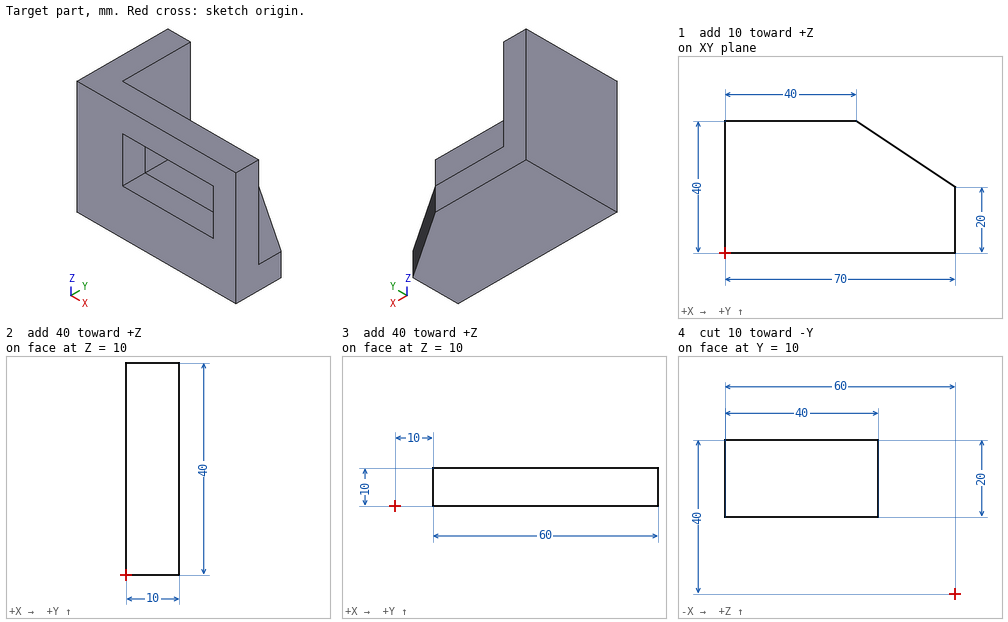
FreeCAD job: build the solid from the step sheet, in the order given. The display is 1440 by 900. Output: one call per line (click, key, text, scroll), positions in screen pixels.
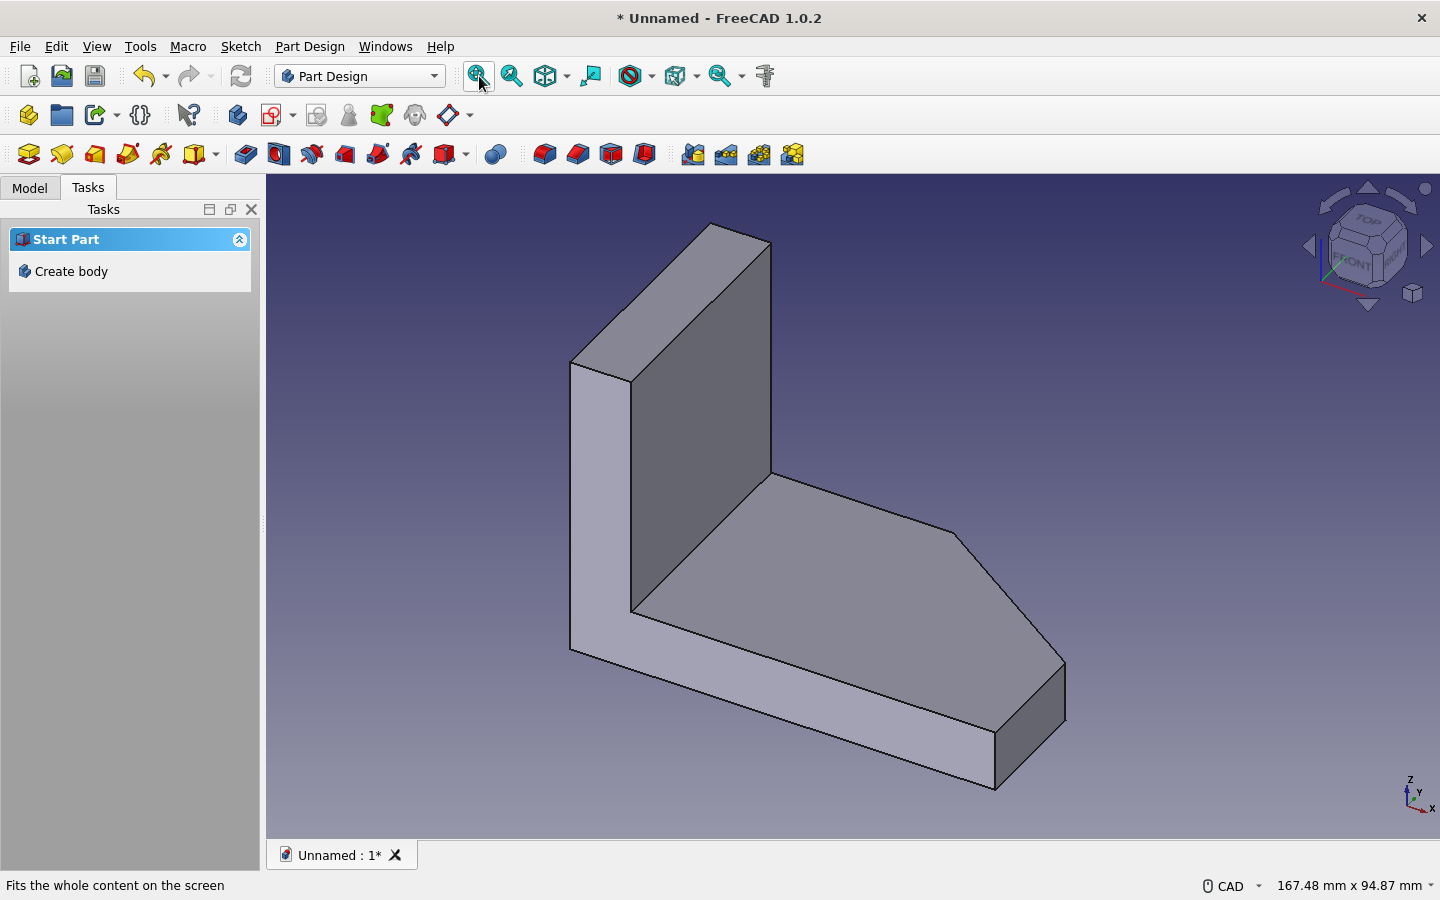
click(831, 584)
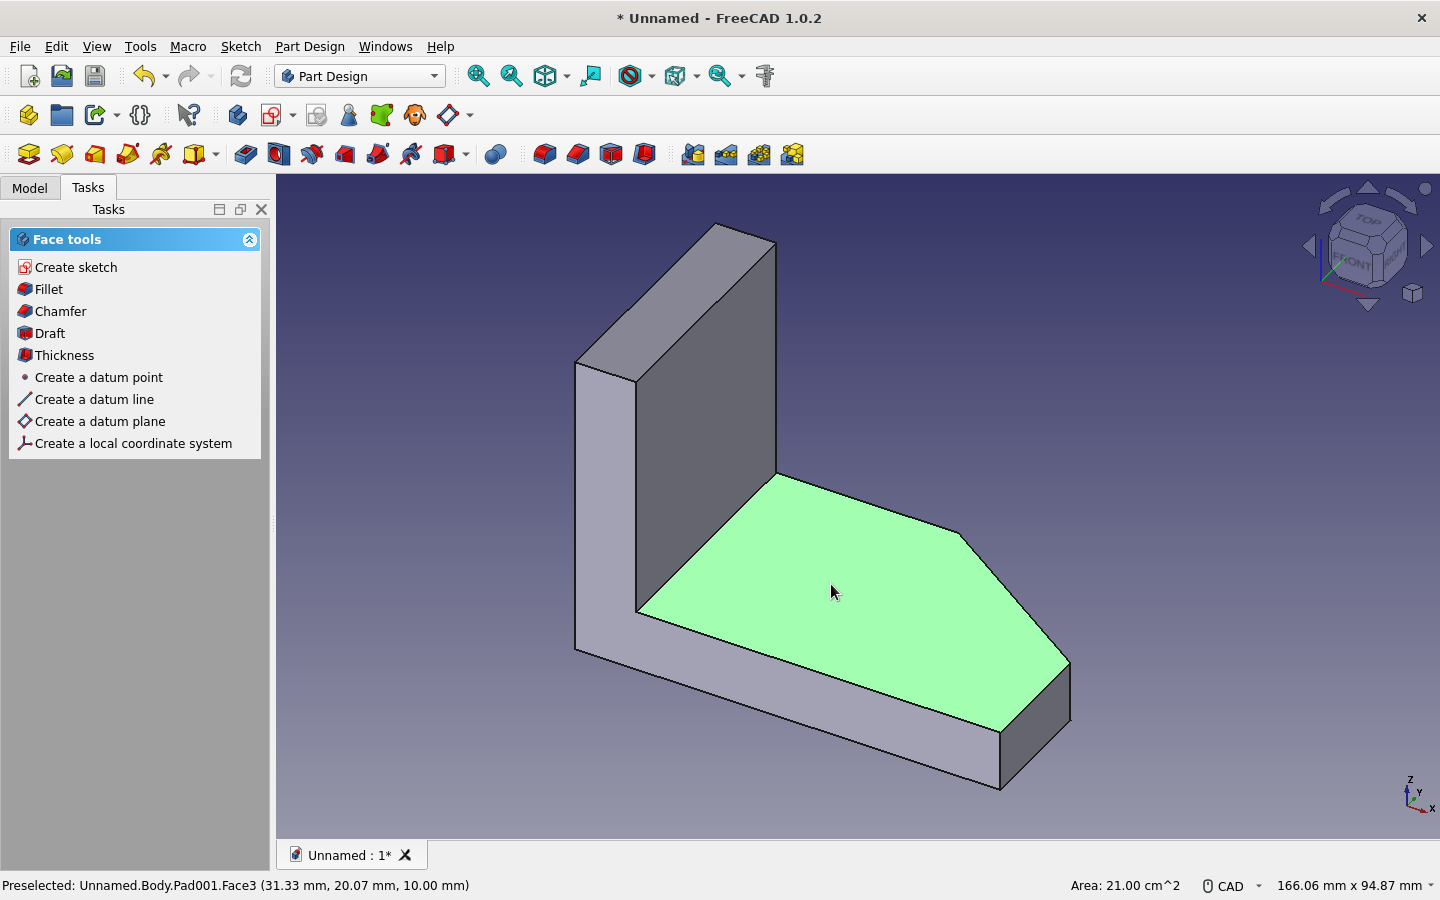
click(270, 116)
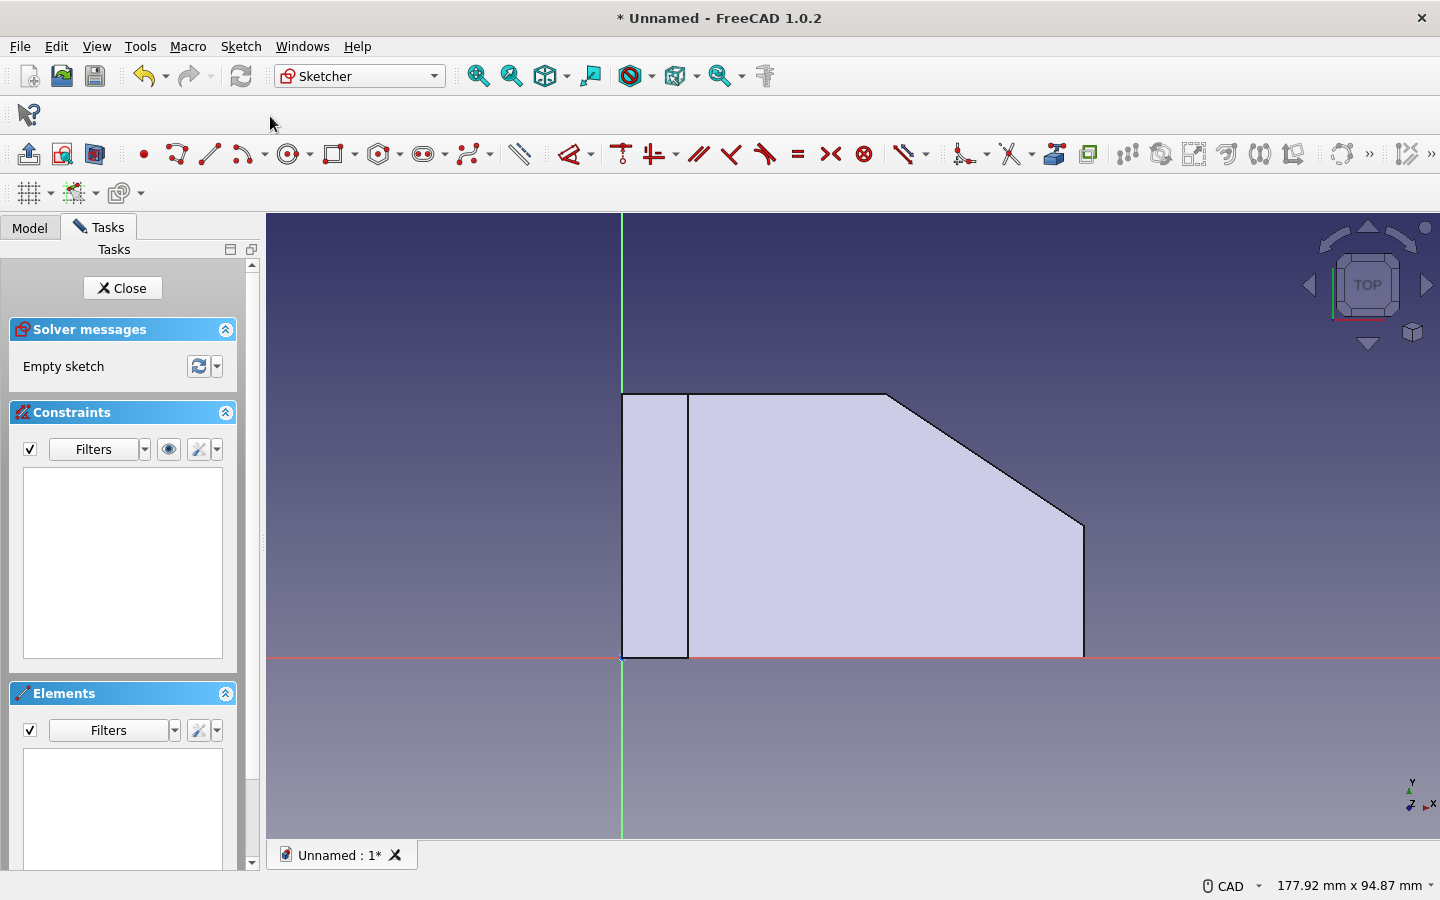
scroll(992, 811, up, 2)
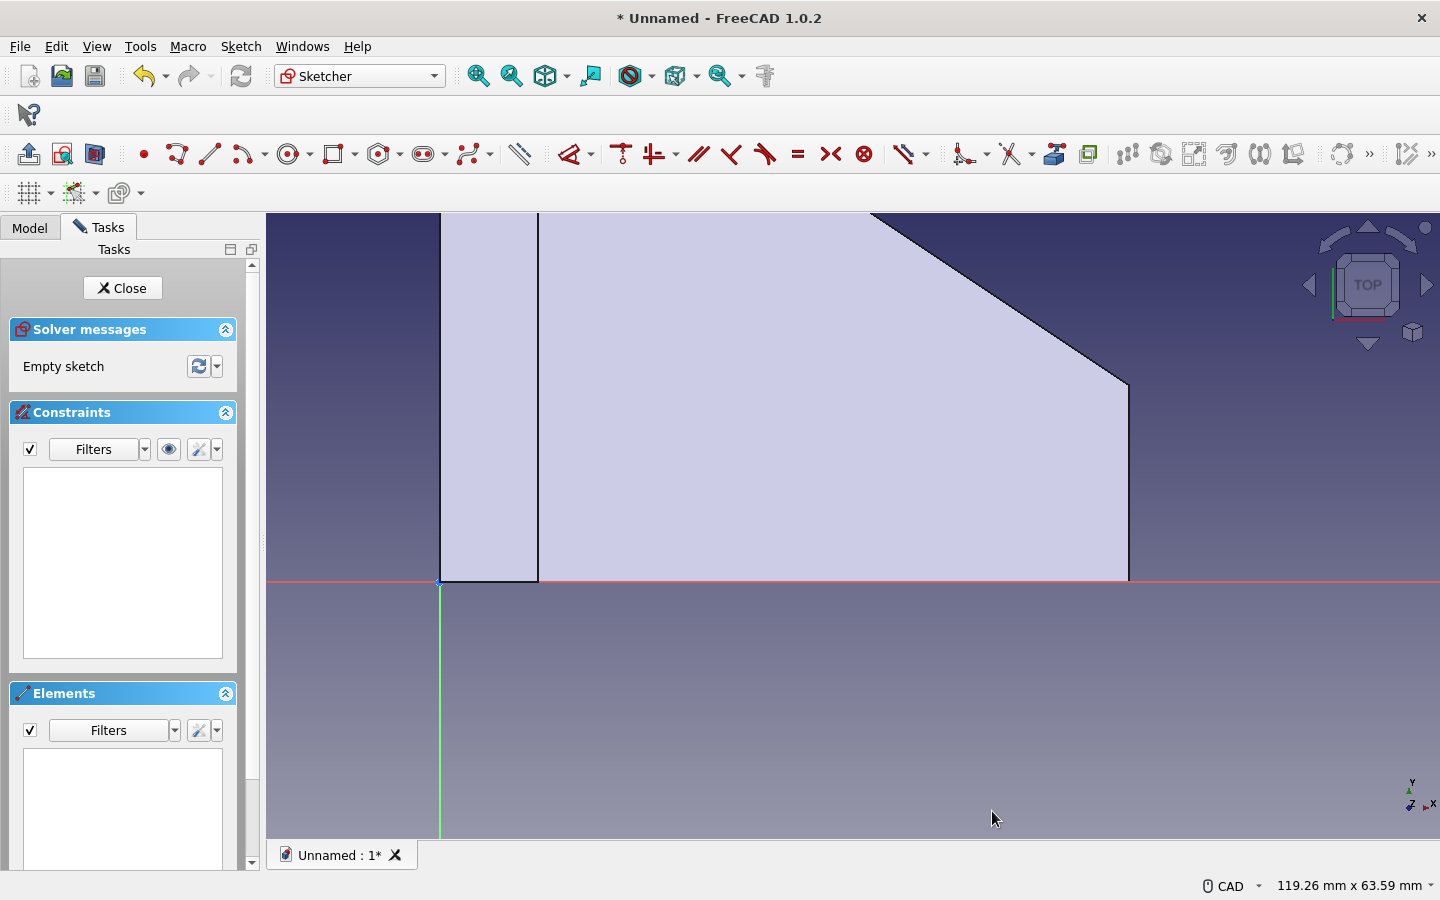
click(332, 154)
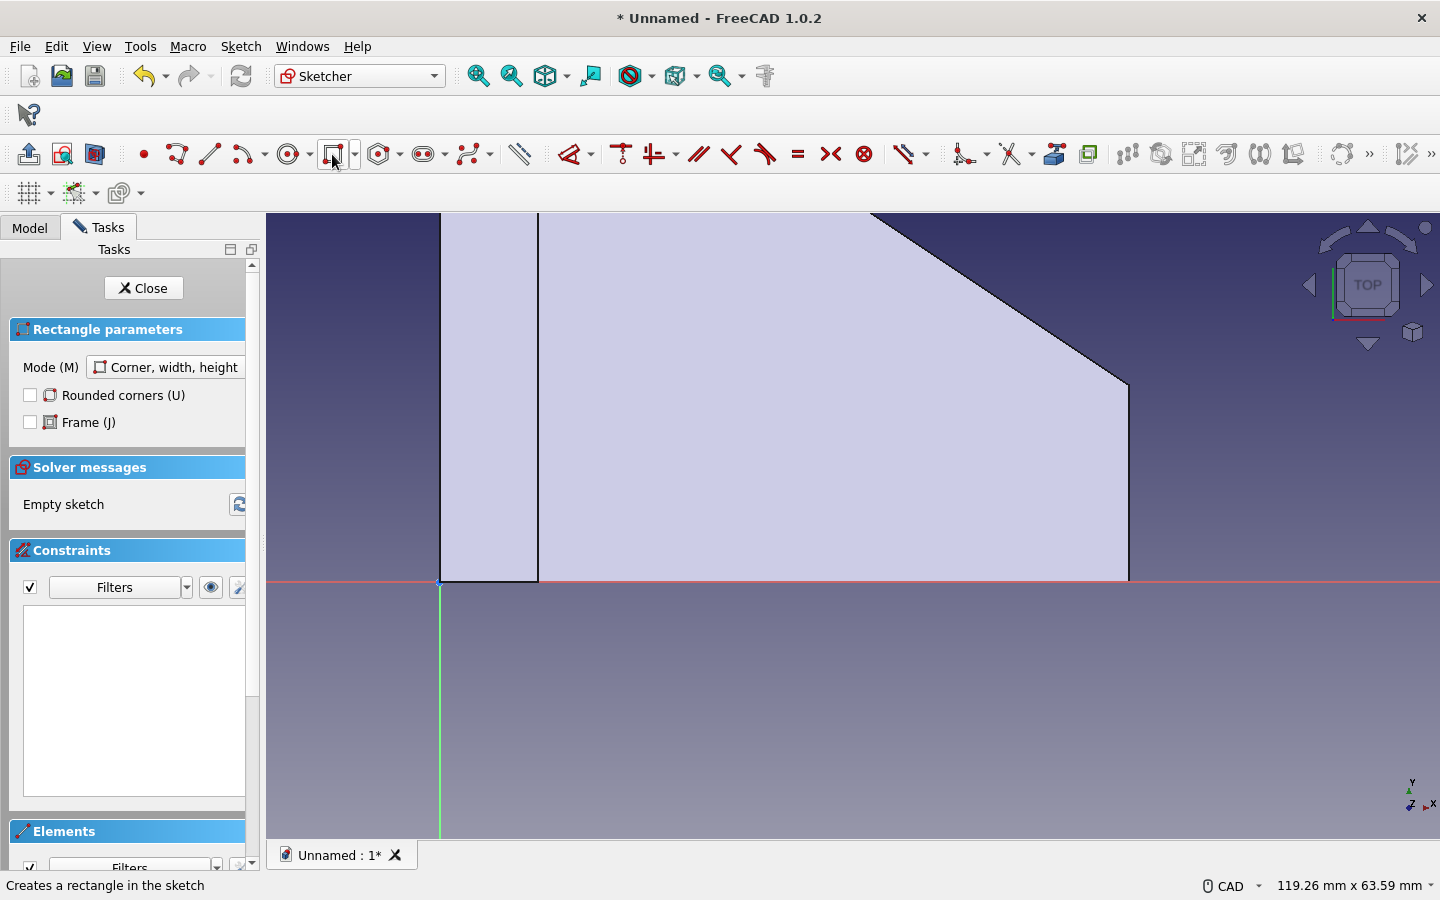
click(538, 484)
click(1129, 582)
key(Escape)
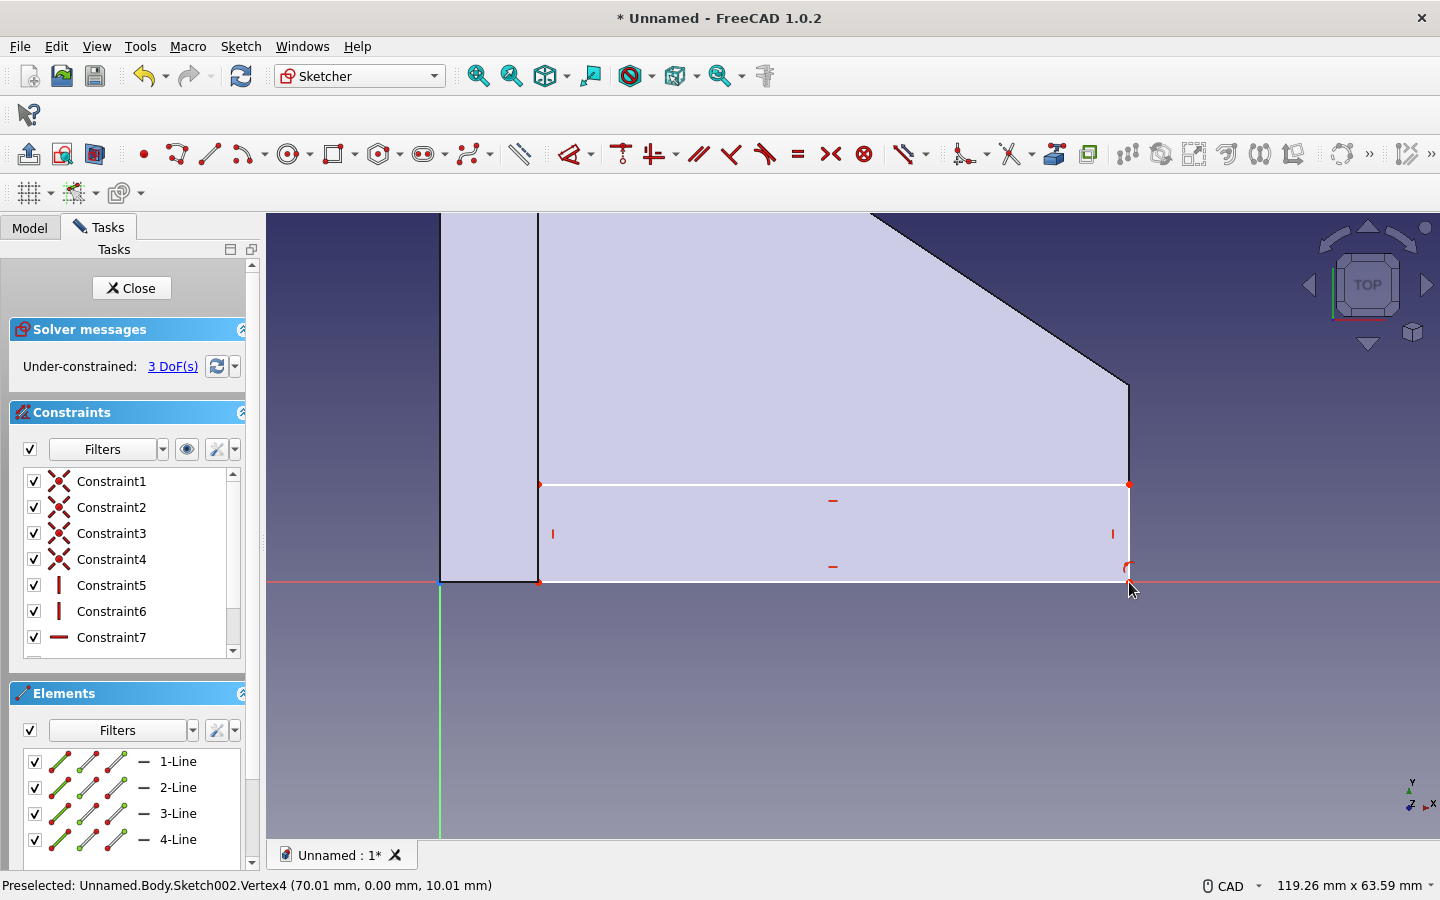
key(d)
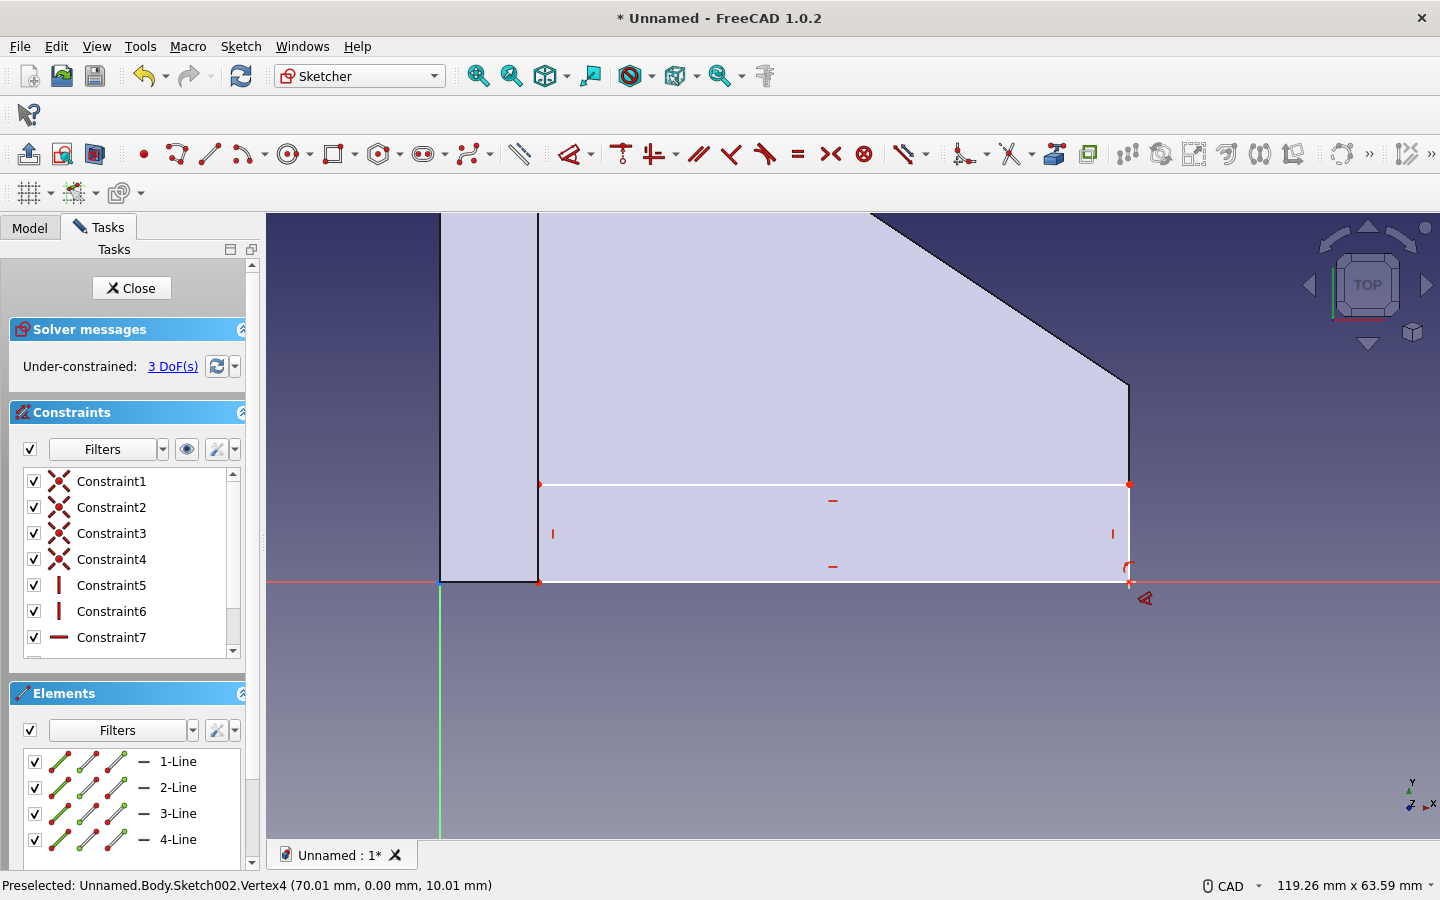
click(538, 514)
click(504, 534)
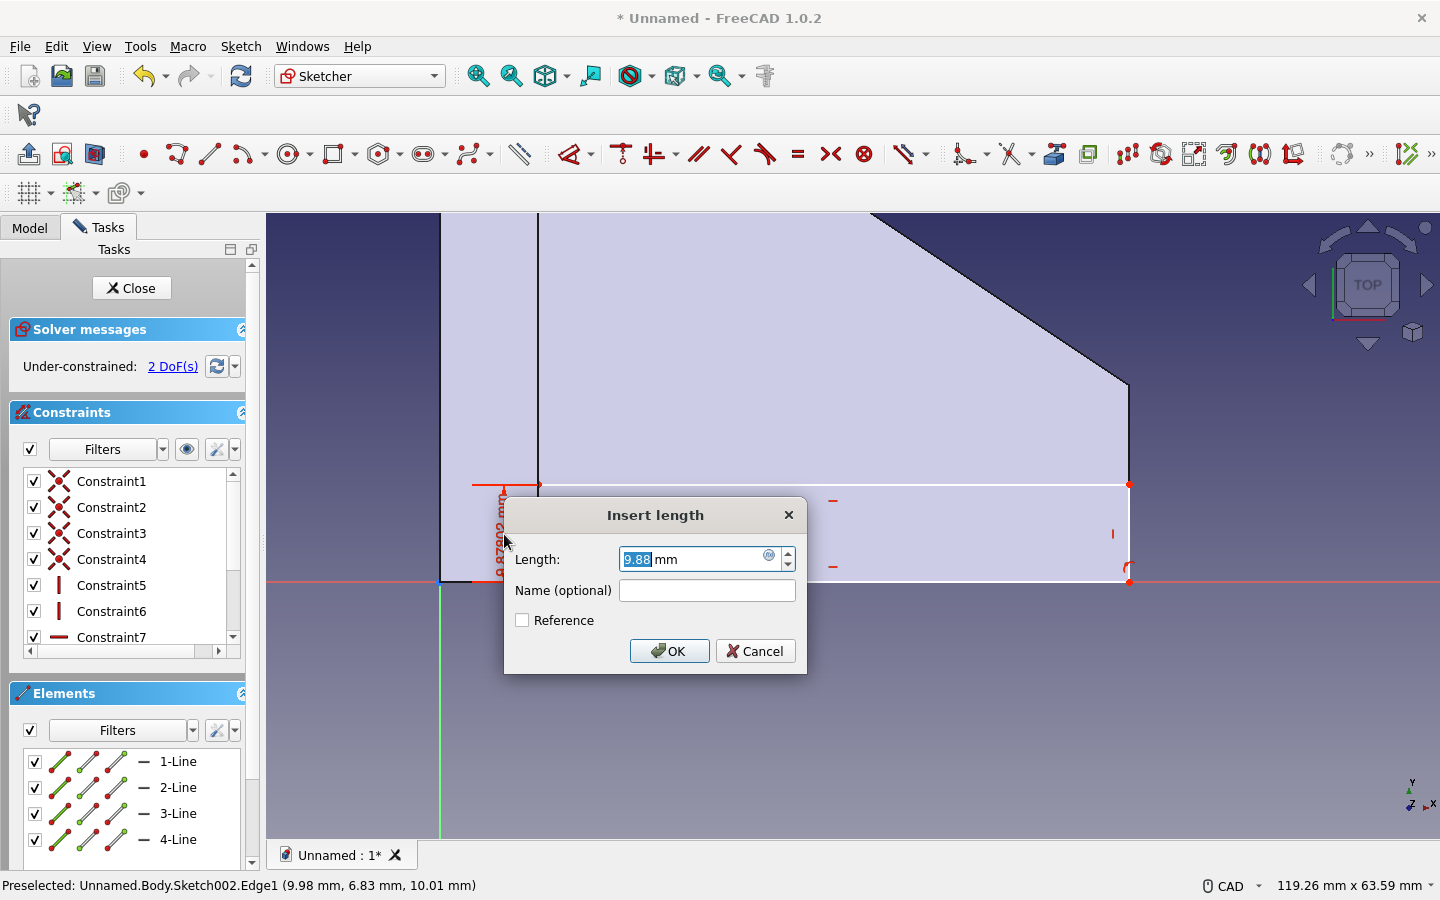
text(10)
key(Return)